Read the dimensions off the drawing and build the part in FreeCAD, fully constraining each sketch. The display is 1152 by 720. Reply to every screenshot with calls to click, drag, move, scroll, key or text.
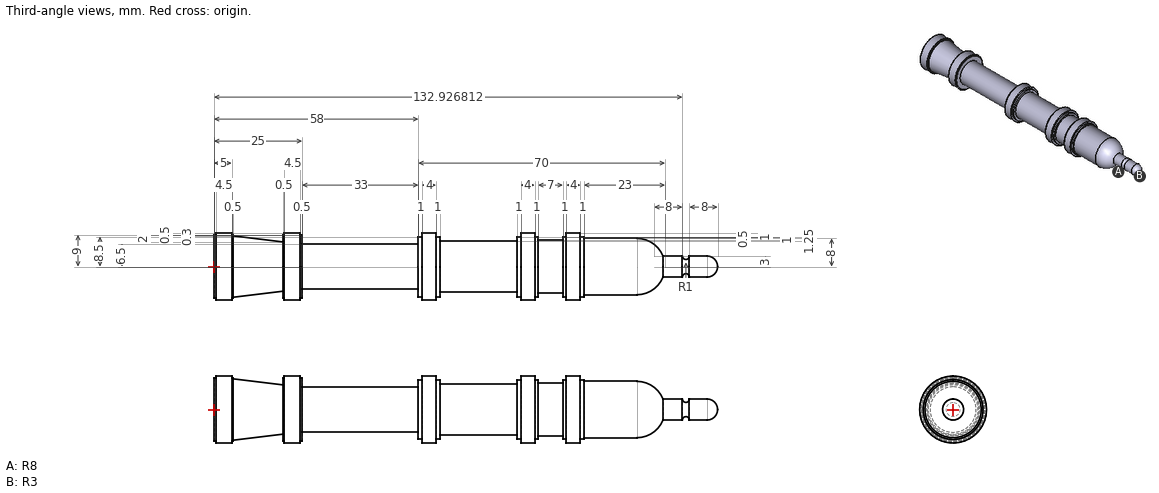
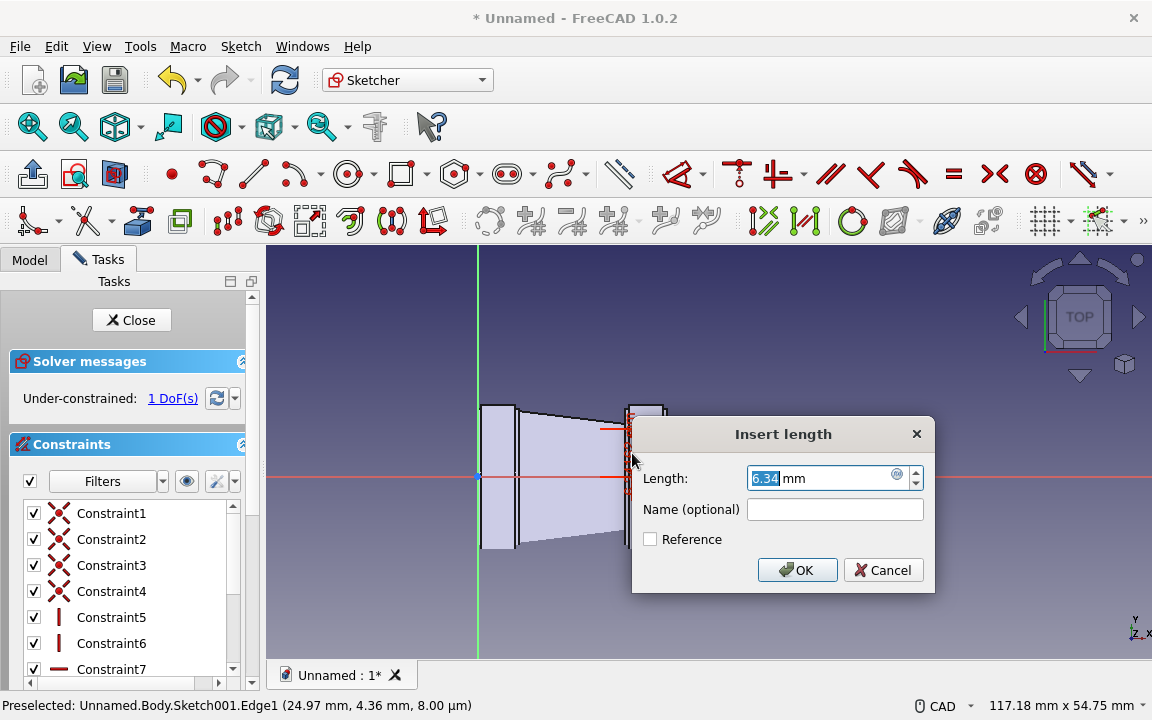
text(6.5)
key(Return)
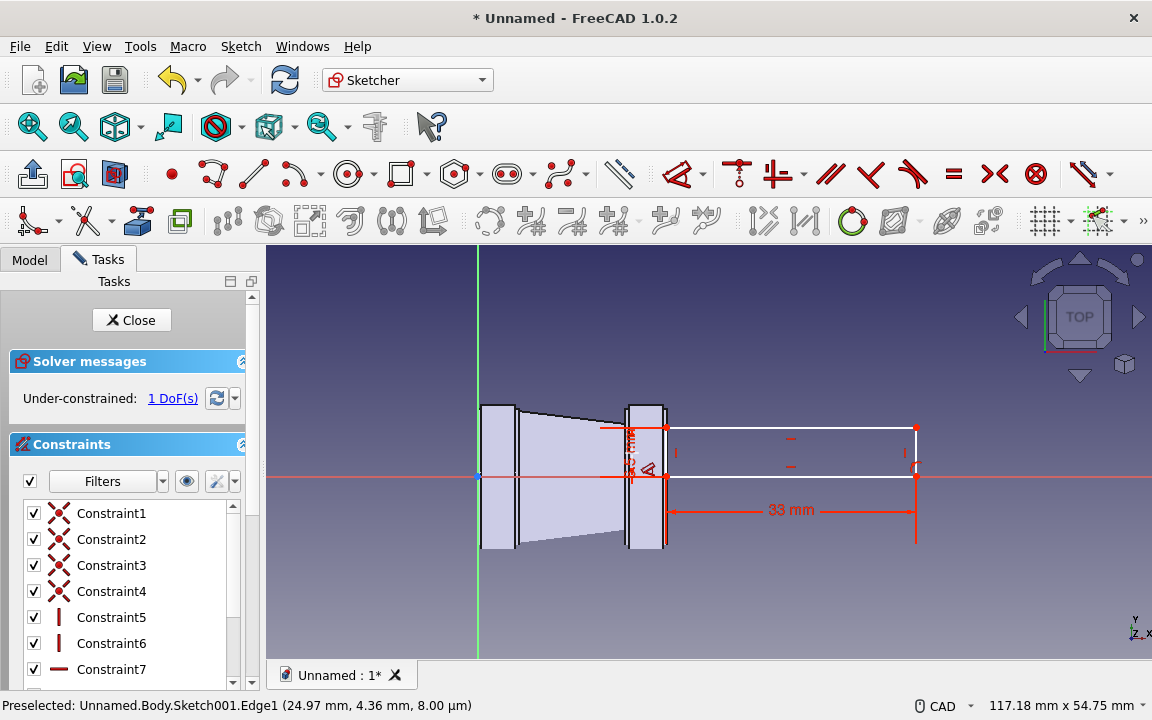
click(666, 428)
click(572, 511)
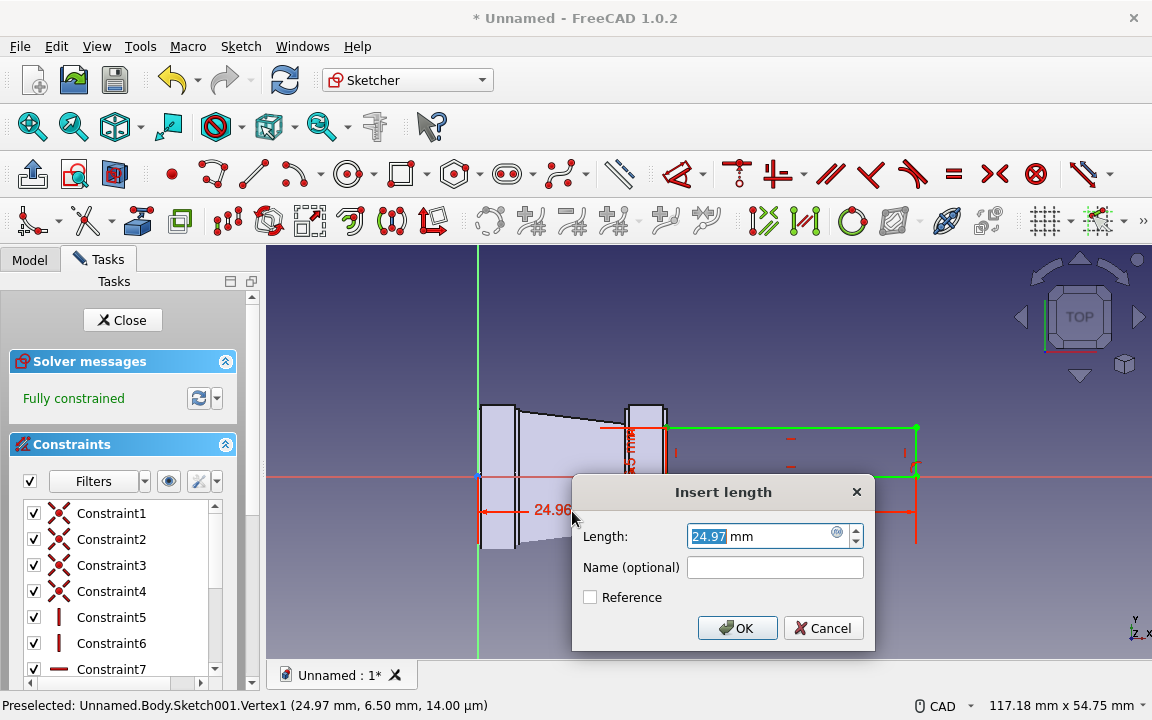
text(25)
key(Return)
key(Escape)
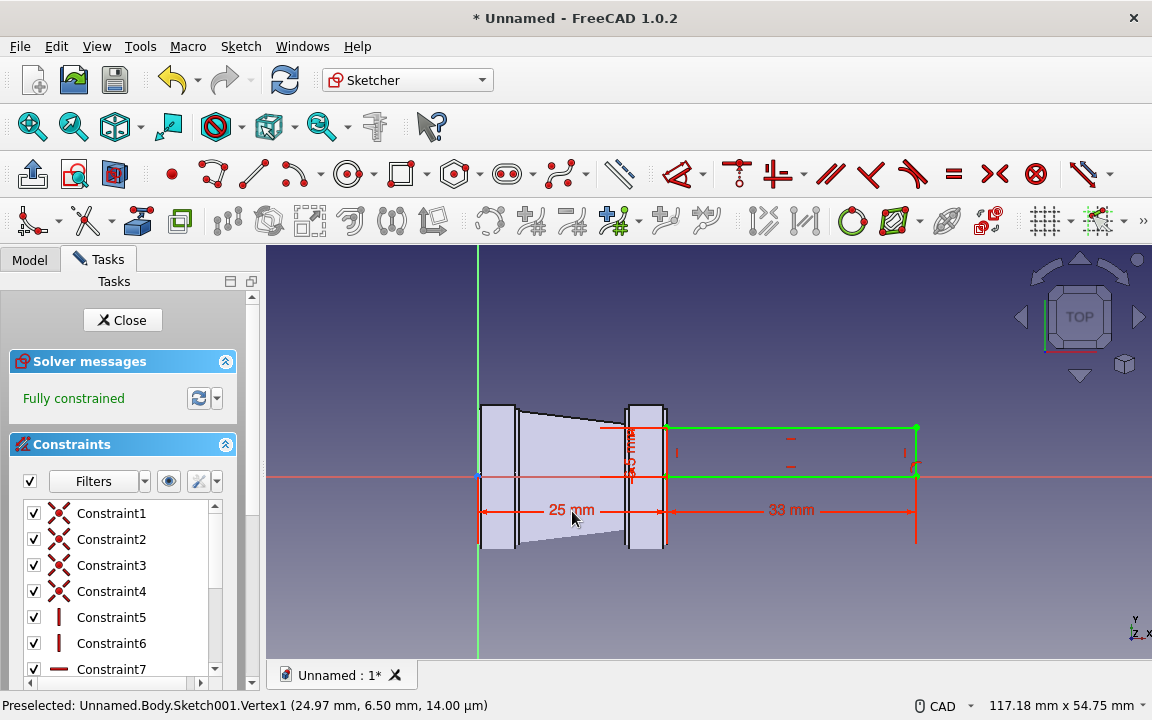
click(123, 320)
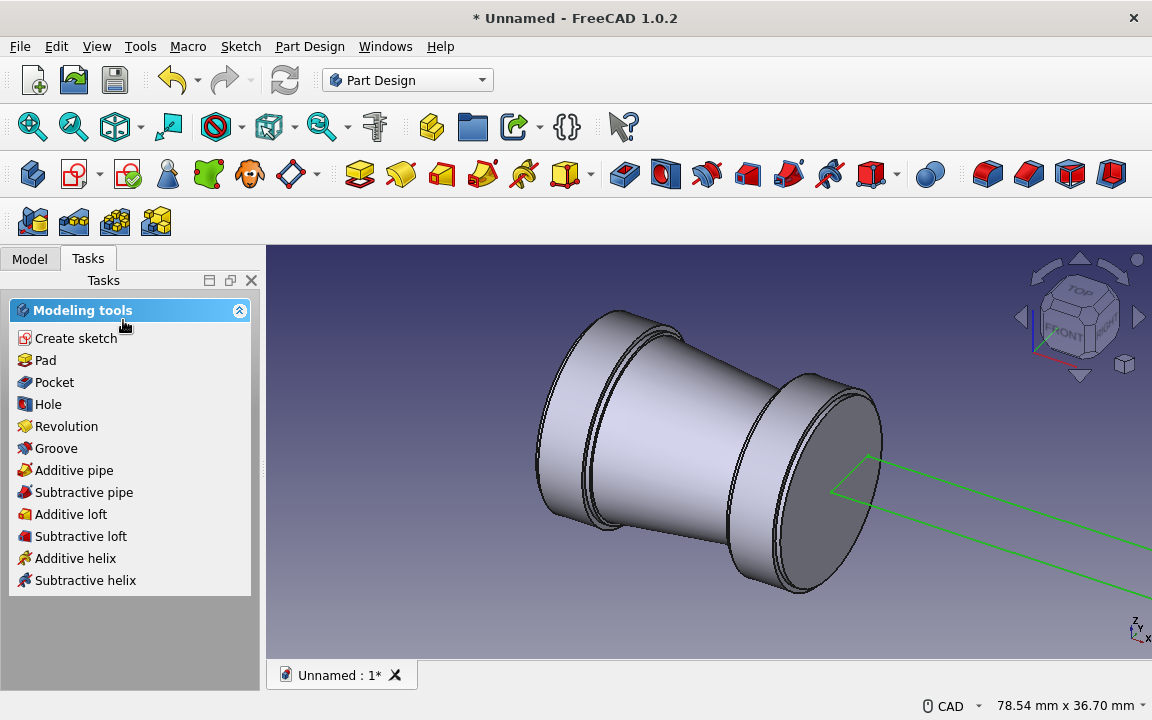
click(401, 174)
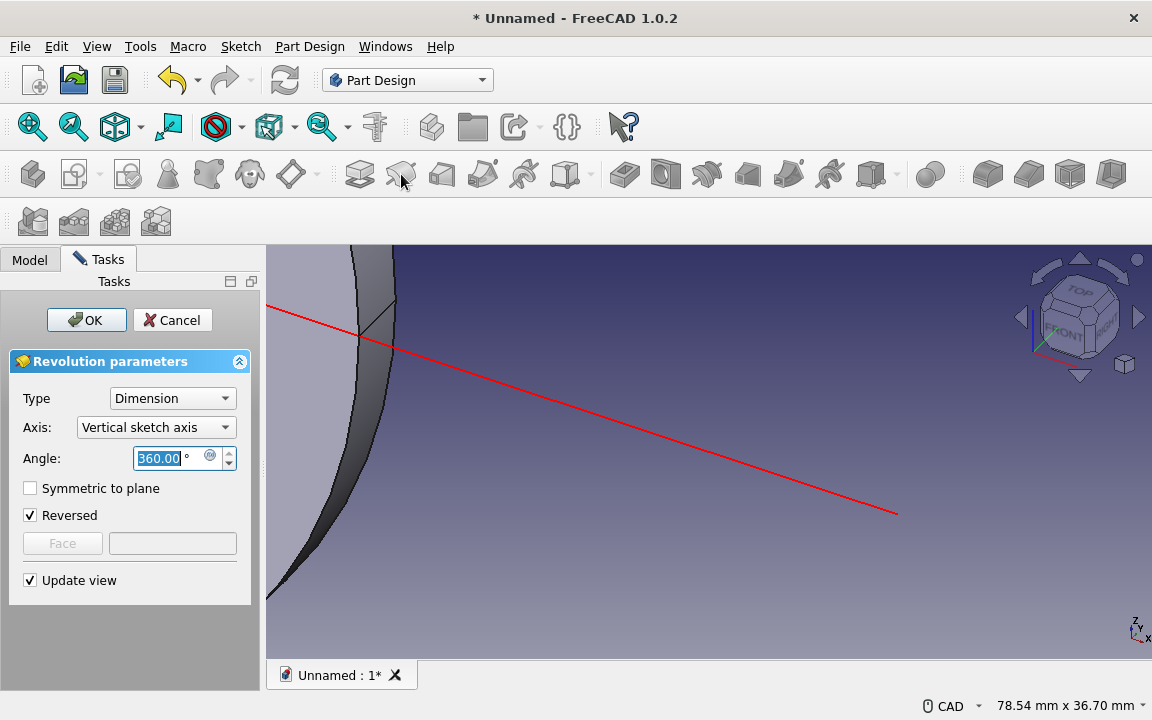
click(157, 428)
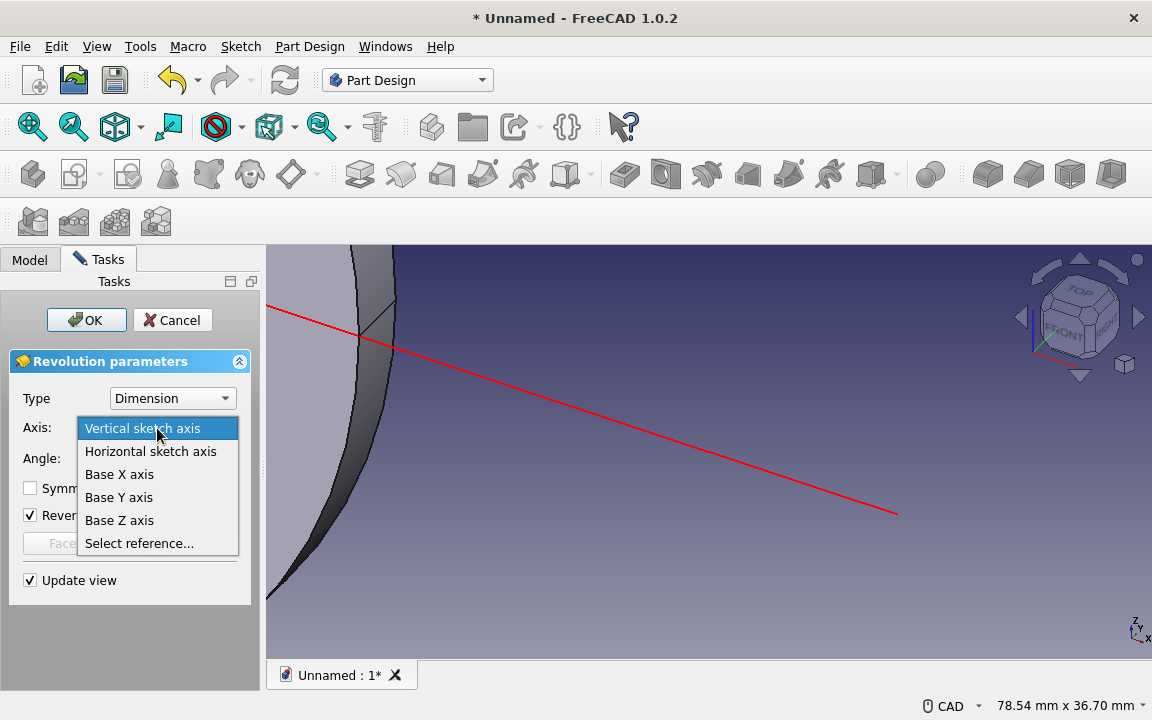
click(156, 452)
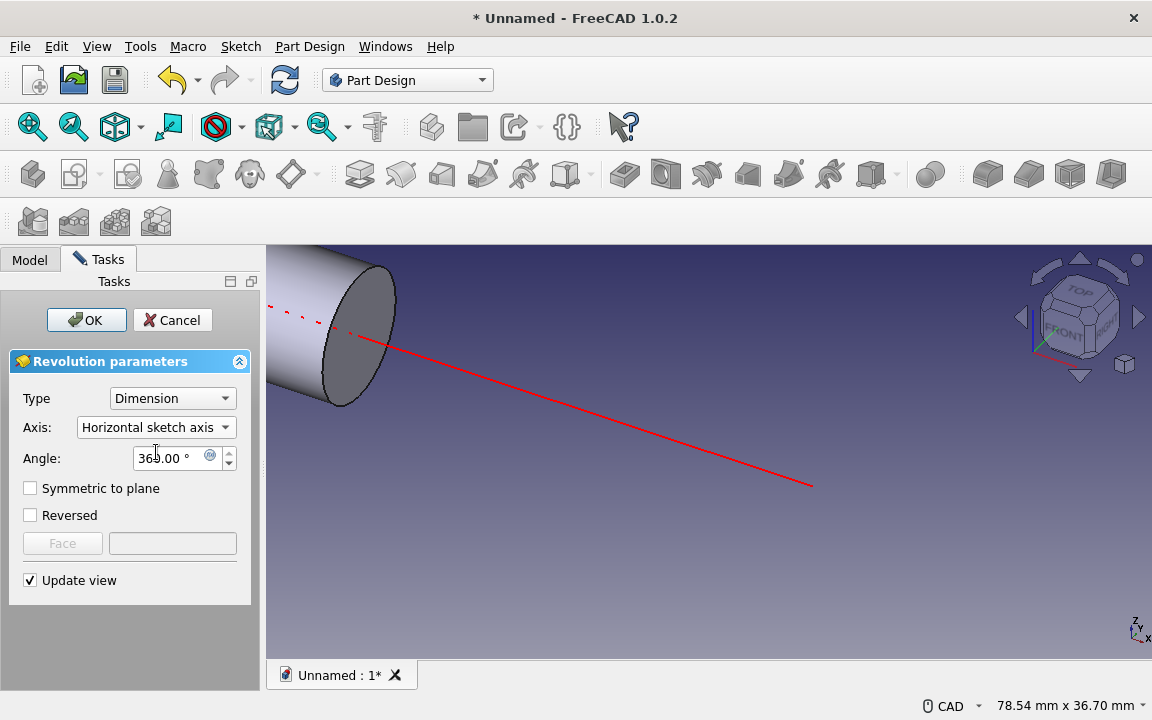
click(87, 320)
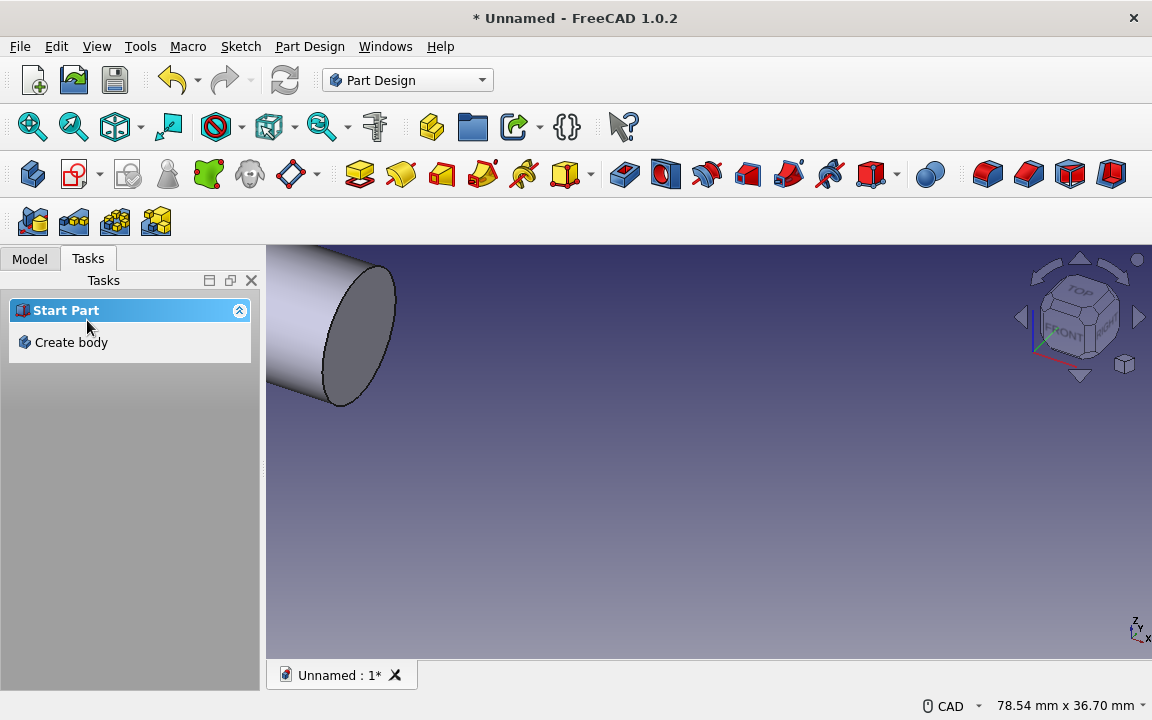
click(33, 128)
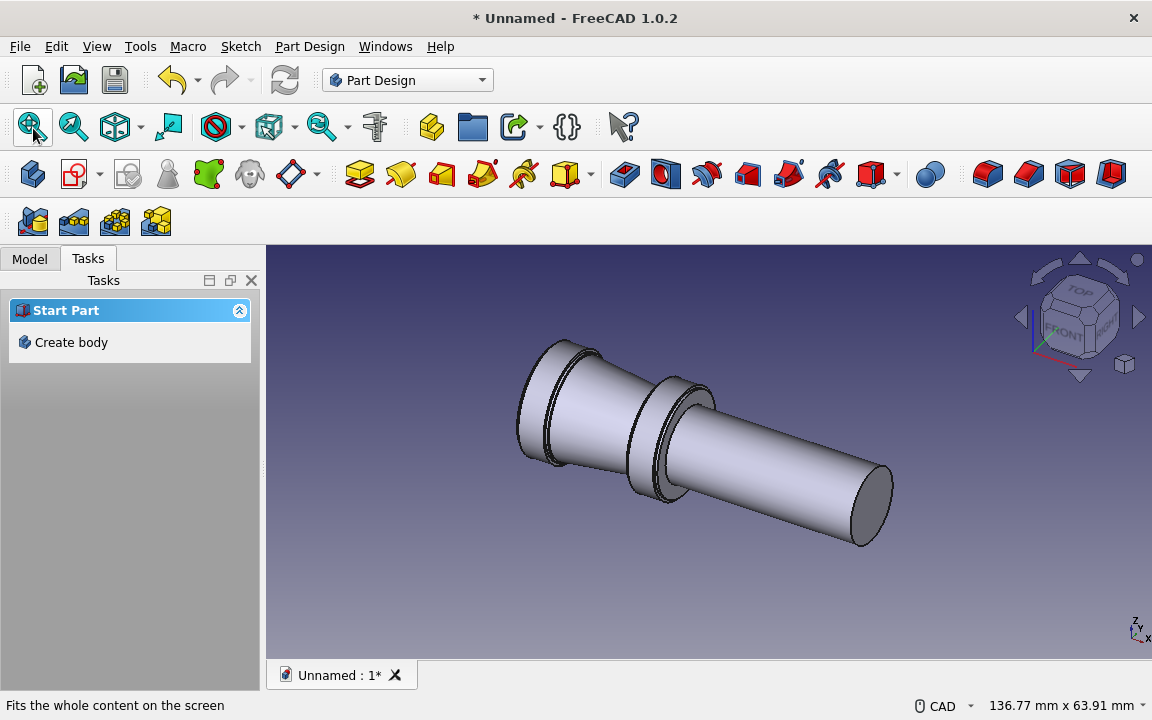
click(74, 174)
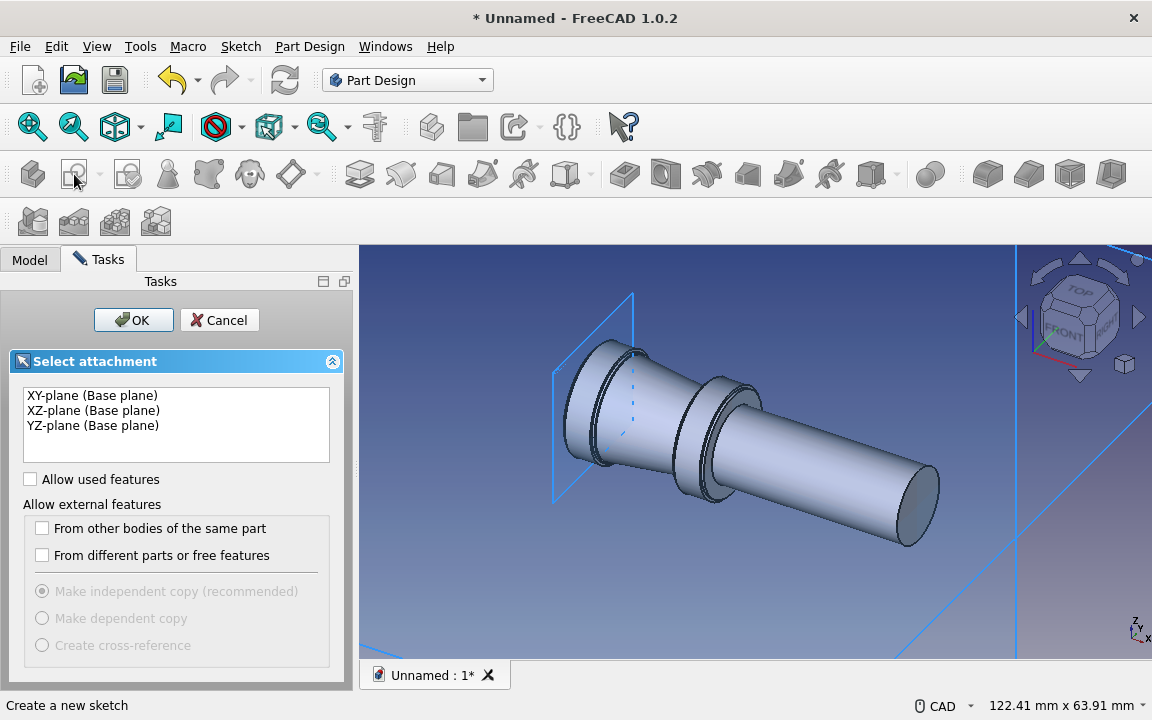
click(84, 396)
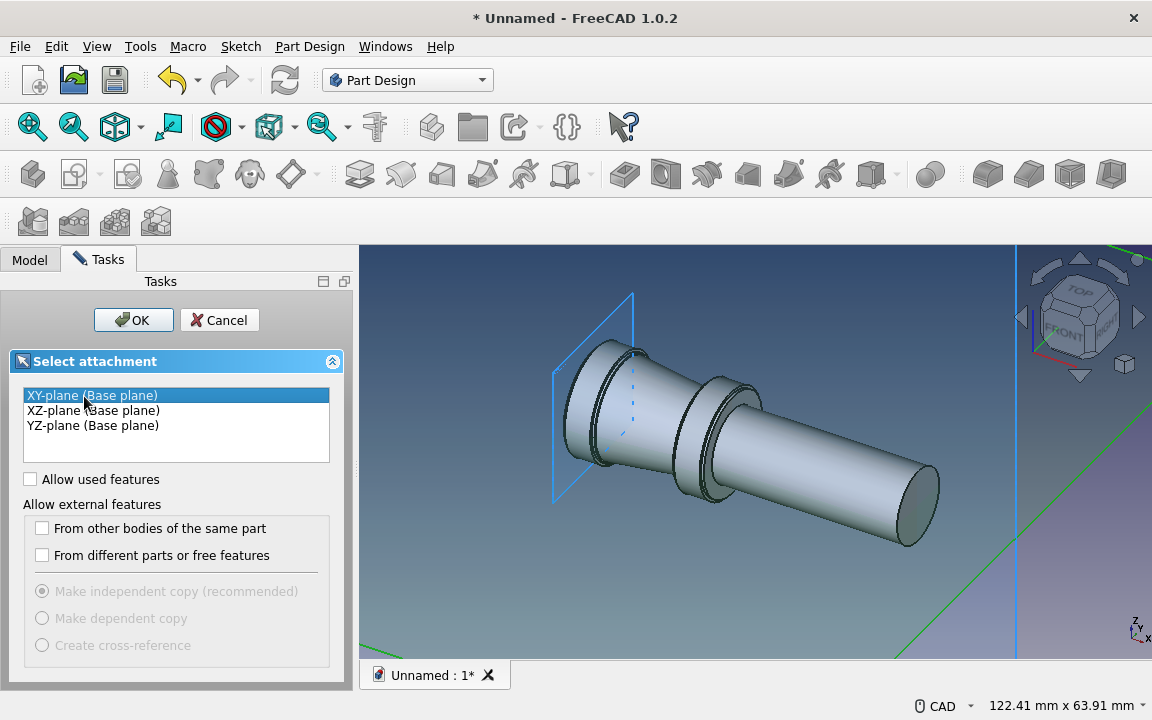
click(134, 320)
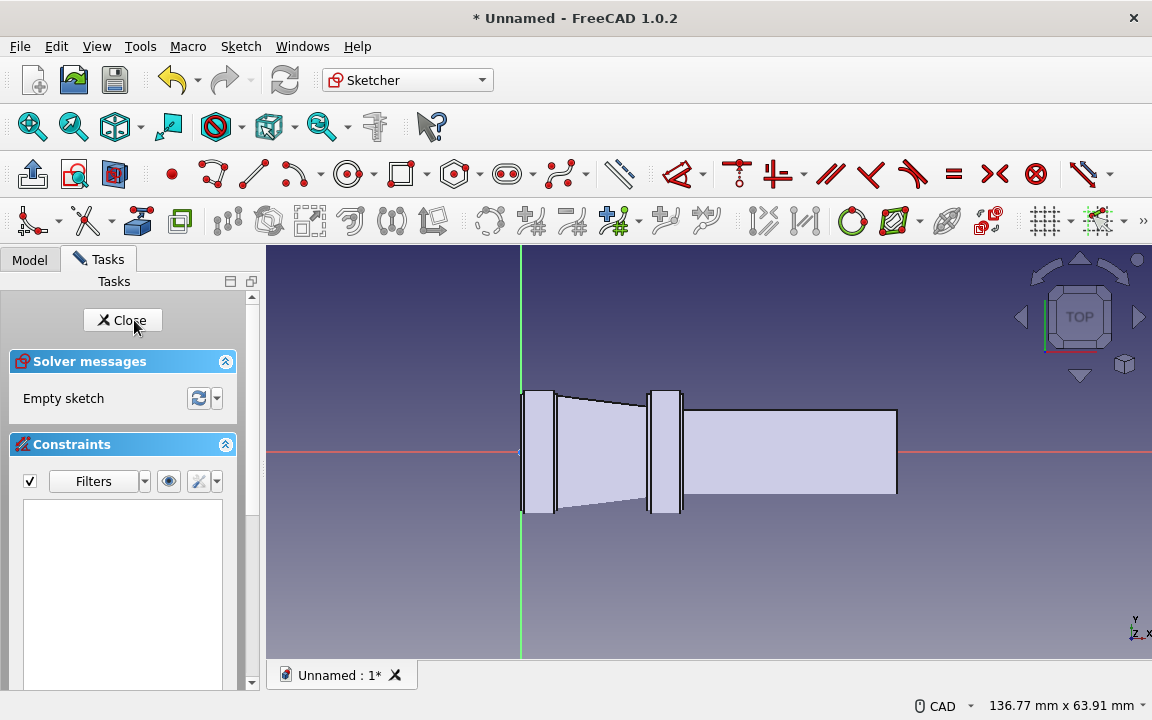
click(115, 174)